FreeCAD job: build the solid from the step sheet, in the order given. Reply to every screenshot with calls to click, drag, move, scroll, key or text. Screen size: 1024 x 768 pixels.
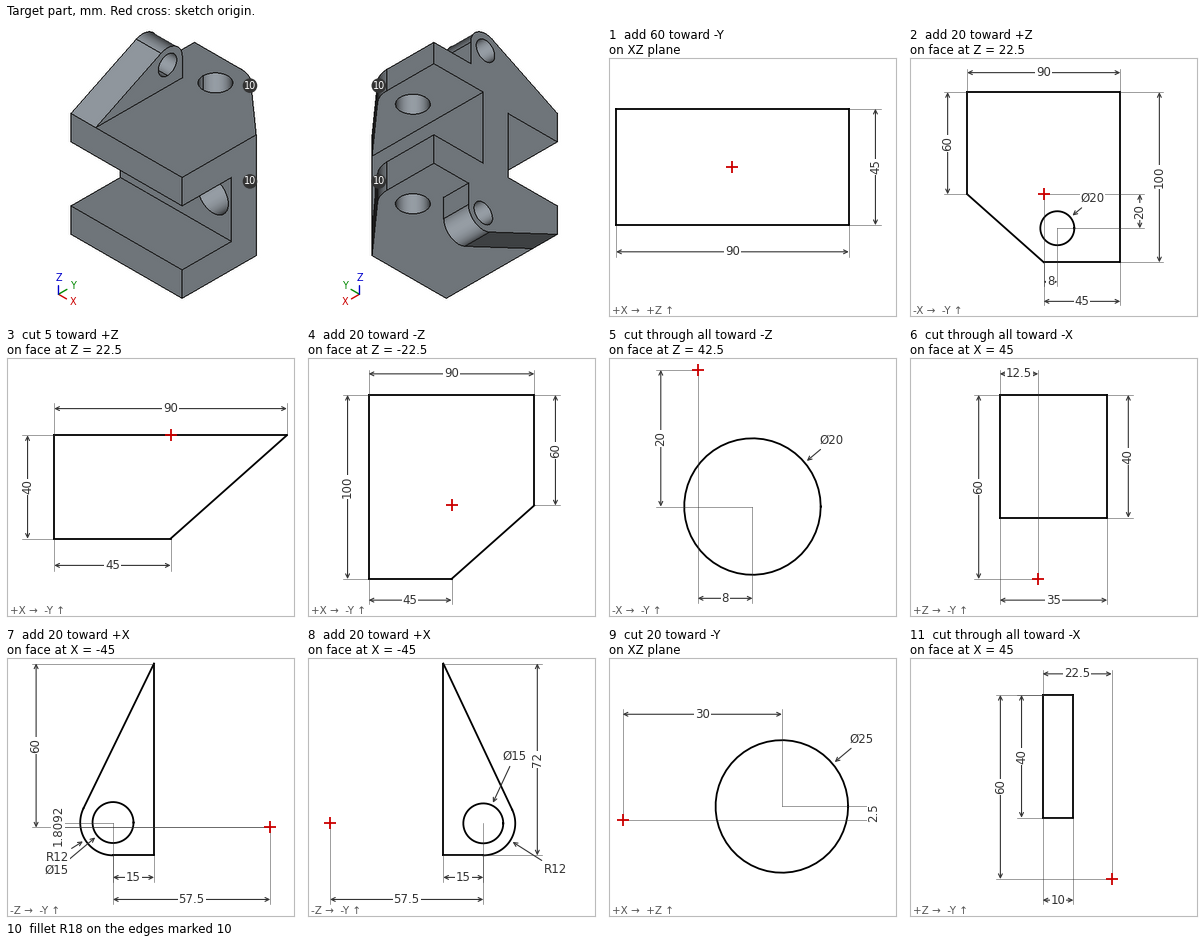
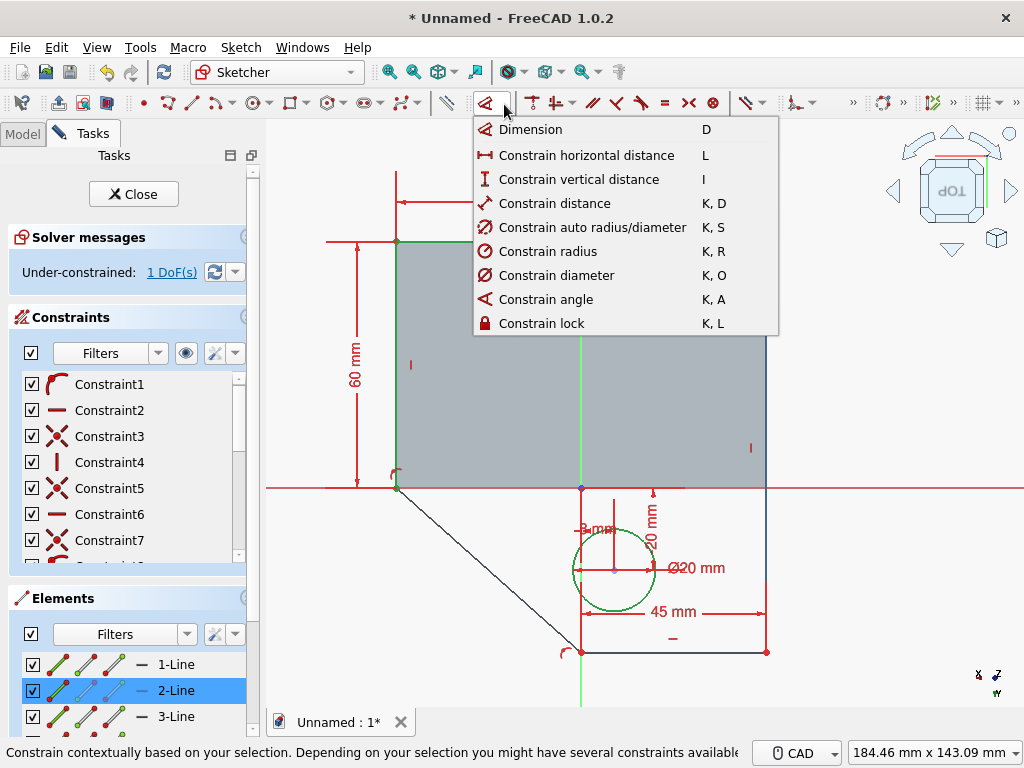
click(626, 179)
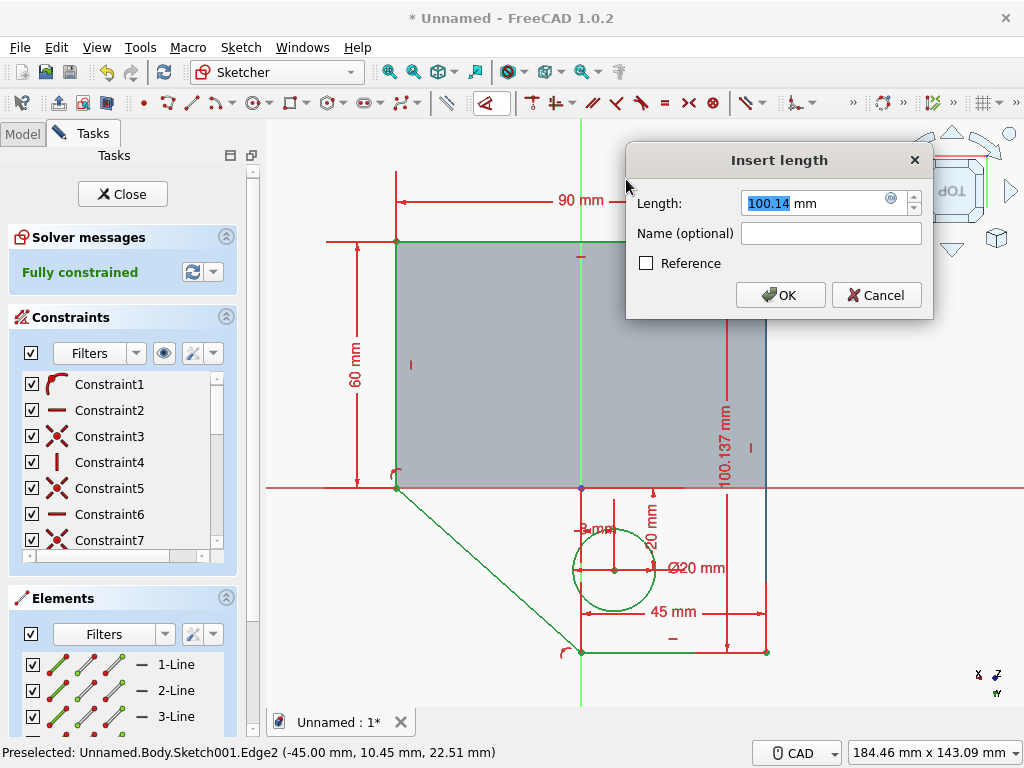
text(100)
key(Return)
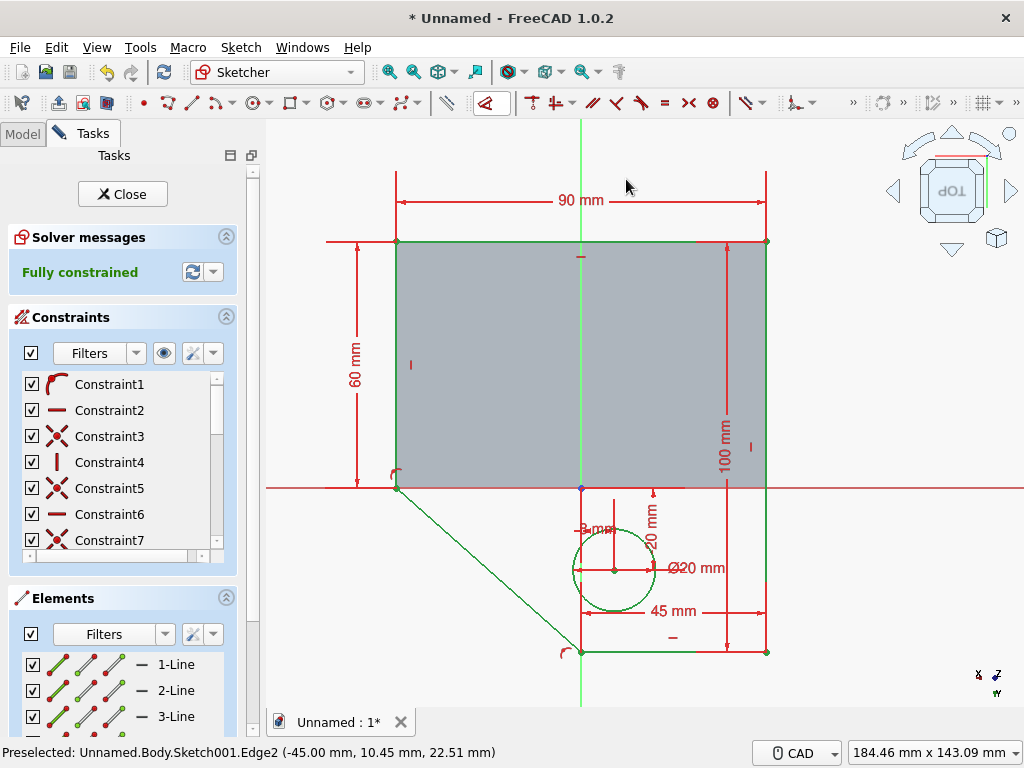
click(123, 194)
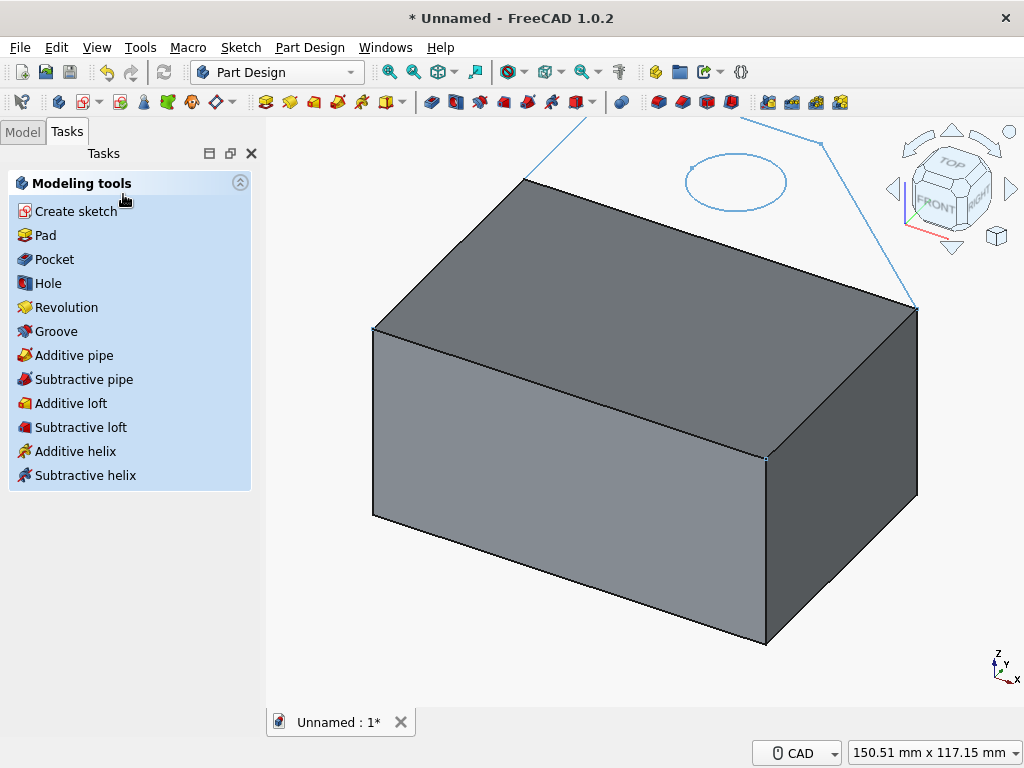
click(266, 102)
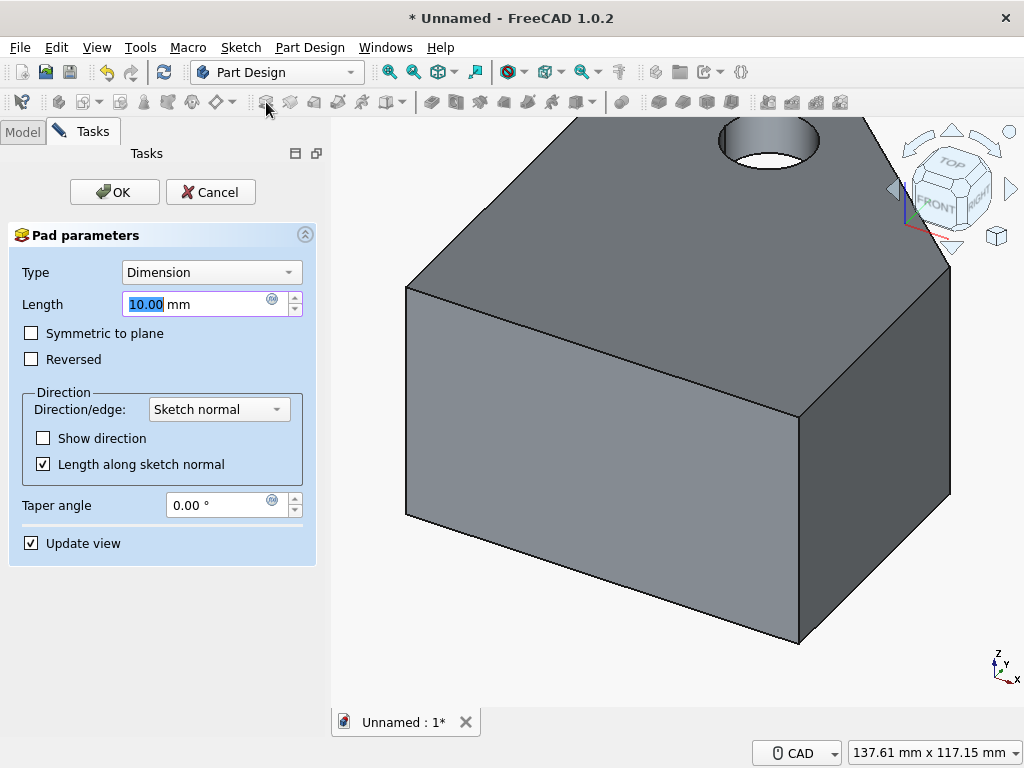
text(20)
key(Tab)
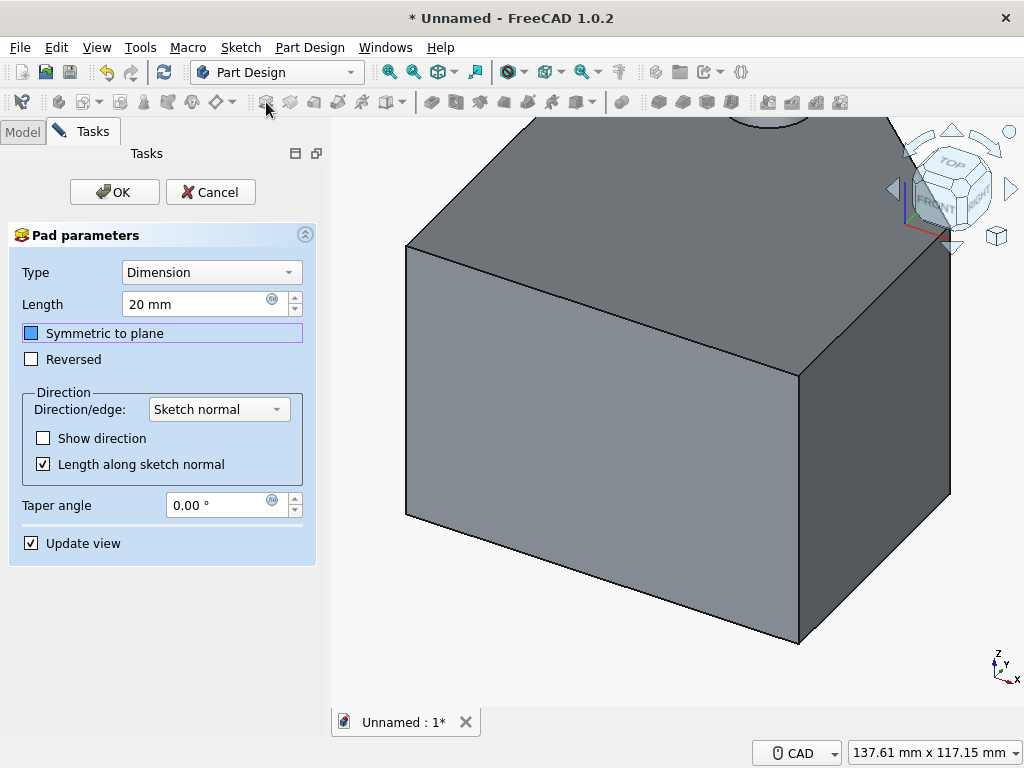
click(115, 192)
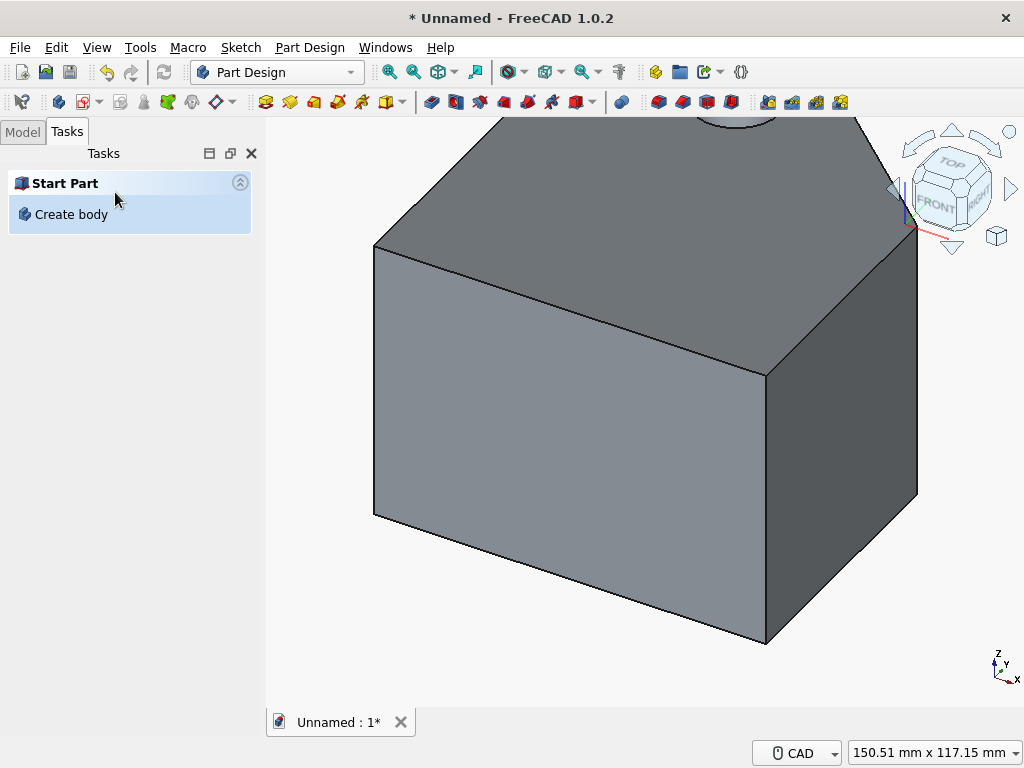
key(v)
key(f)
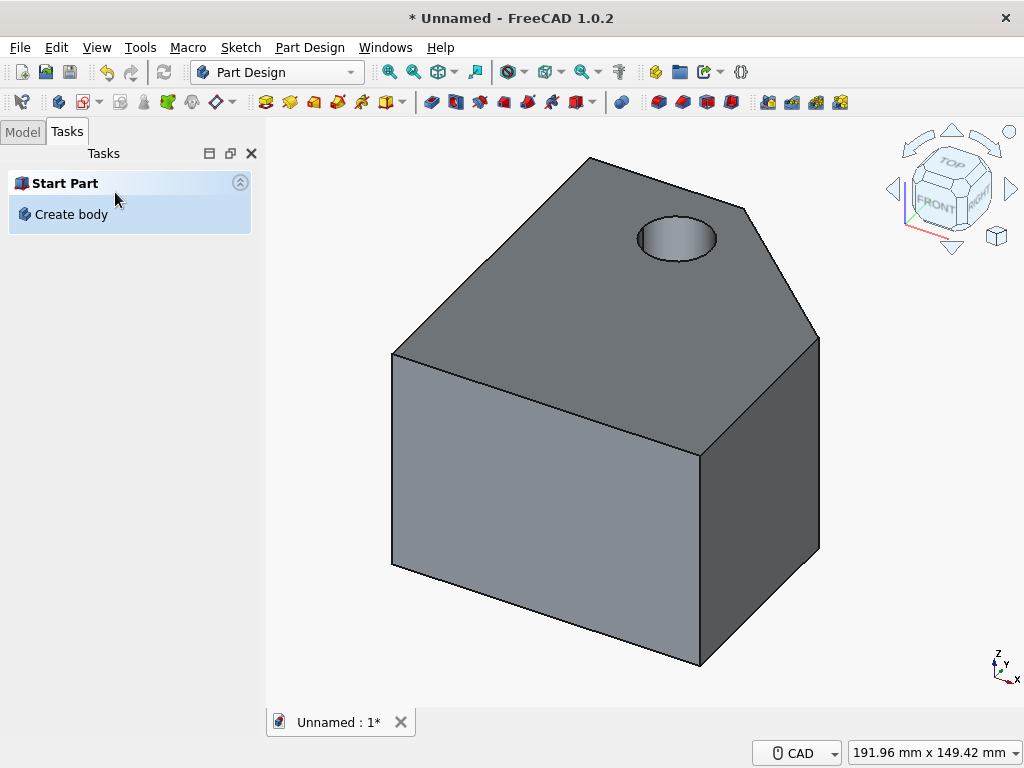
key(5)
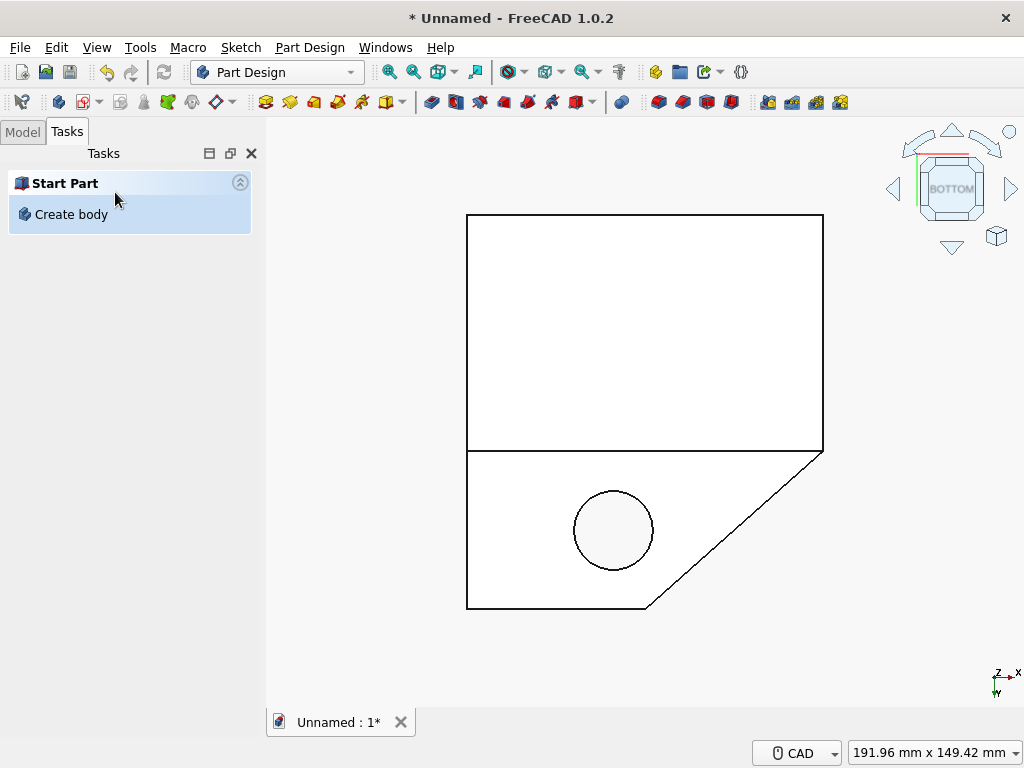
click(696, 507)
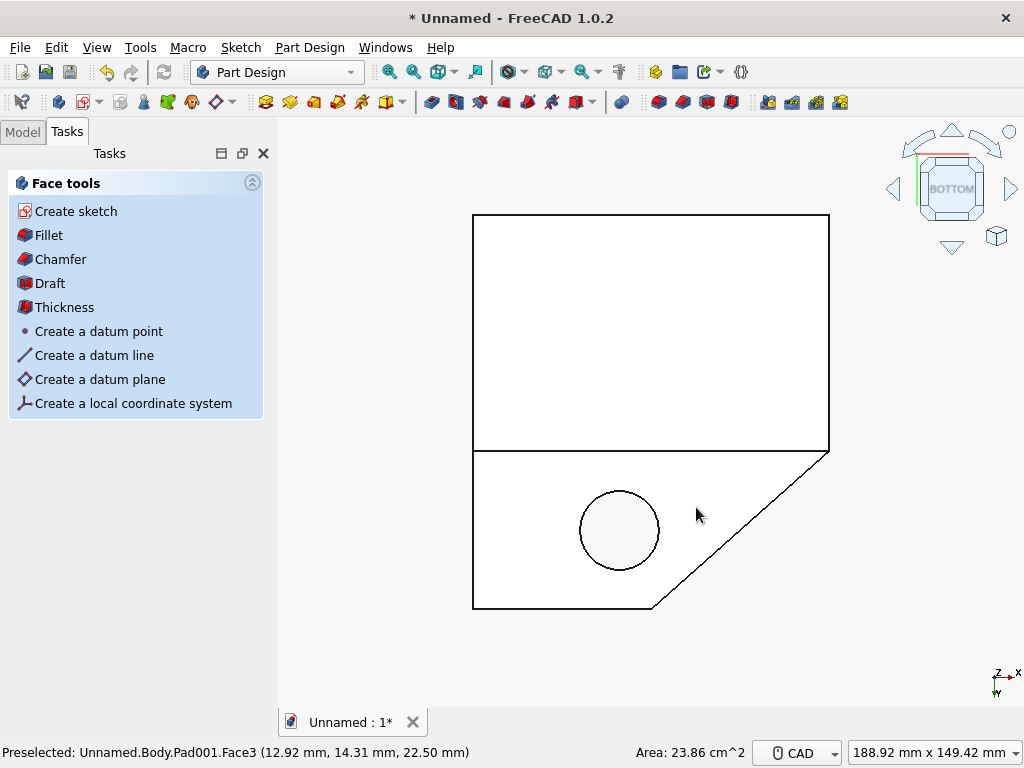
click(84, 102)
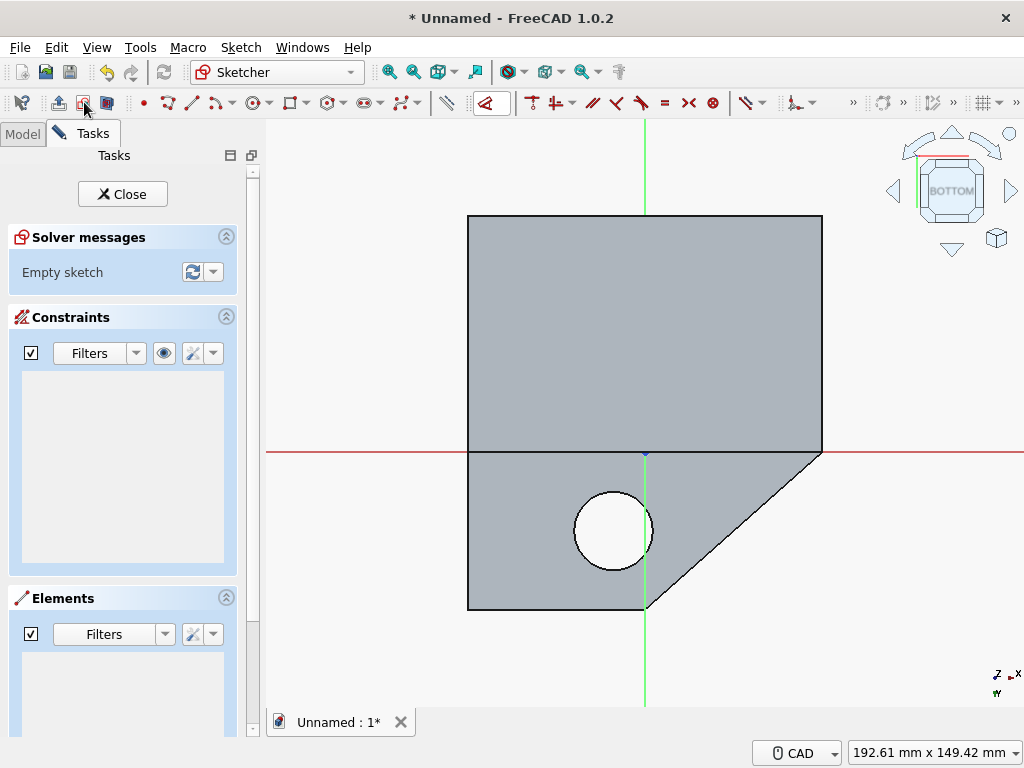
key(q)
key(s)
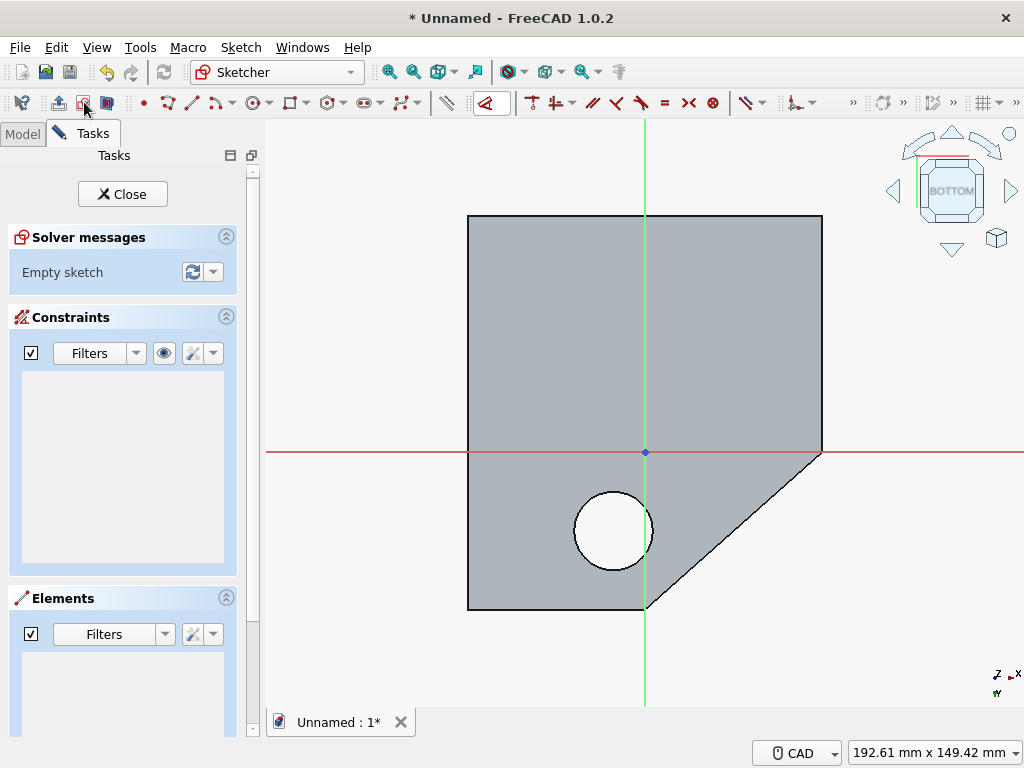
key(g)
key(m)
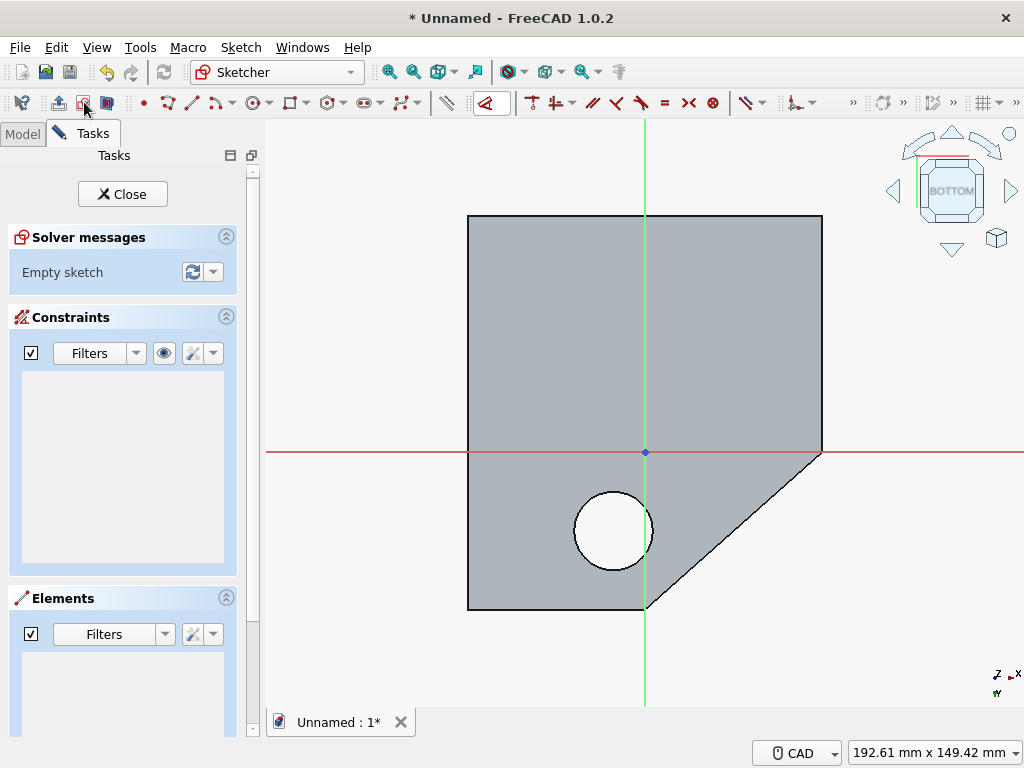
click(645, 610)
click(822, 452)
click(468, 461)
click(468, 610)
click(645, 611)
key(Escape)
key(Escape)